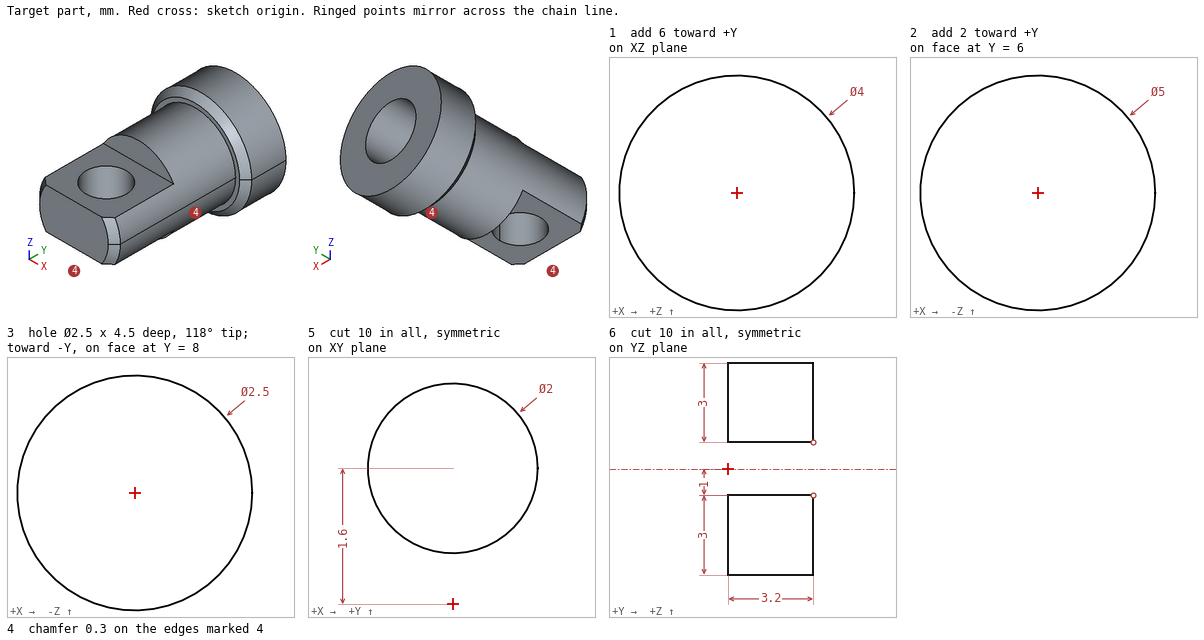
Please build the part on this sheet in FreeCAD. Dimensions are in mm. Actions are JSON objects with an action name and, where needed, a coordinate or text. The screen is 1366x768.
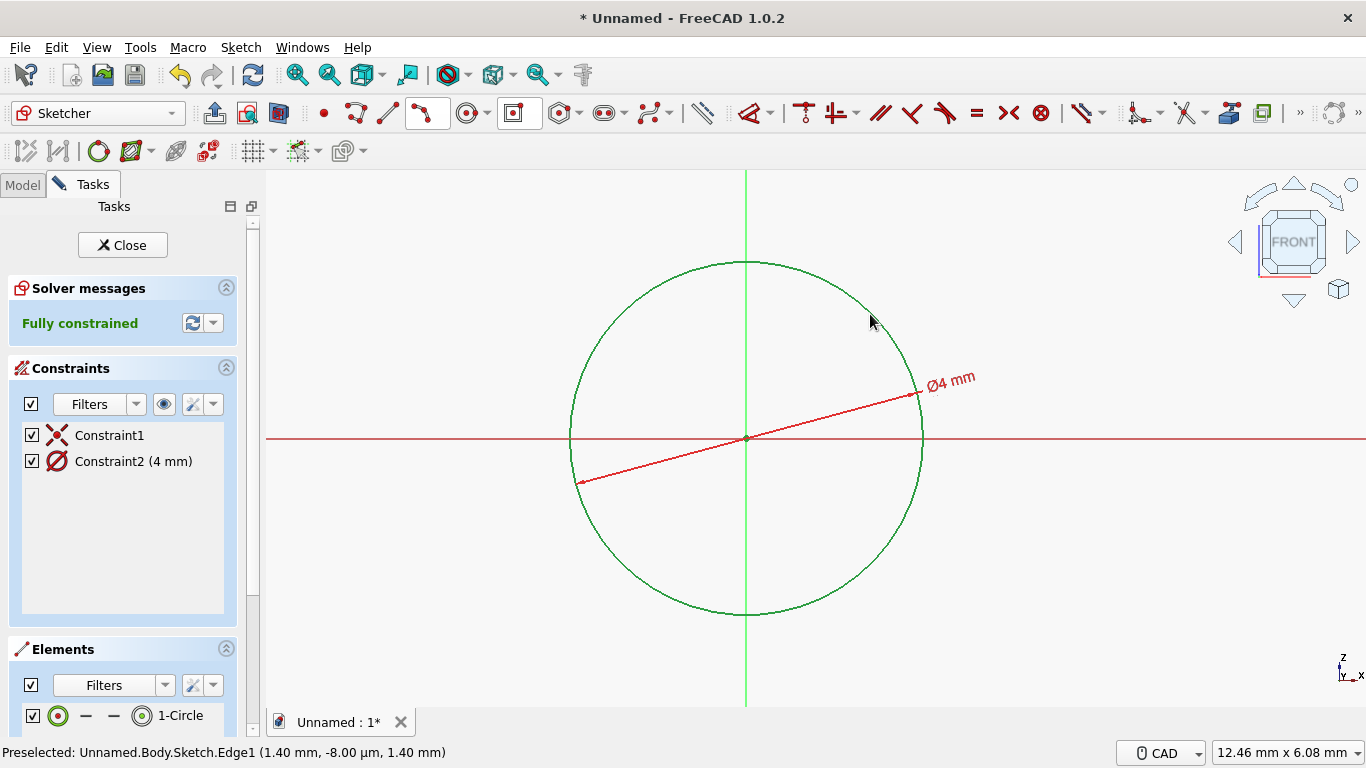
{"action": "left_click", "coordinate": [123, 245]}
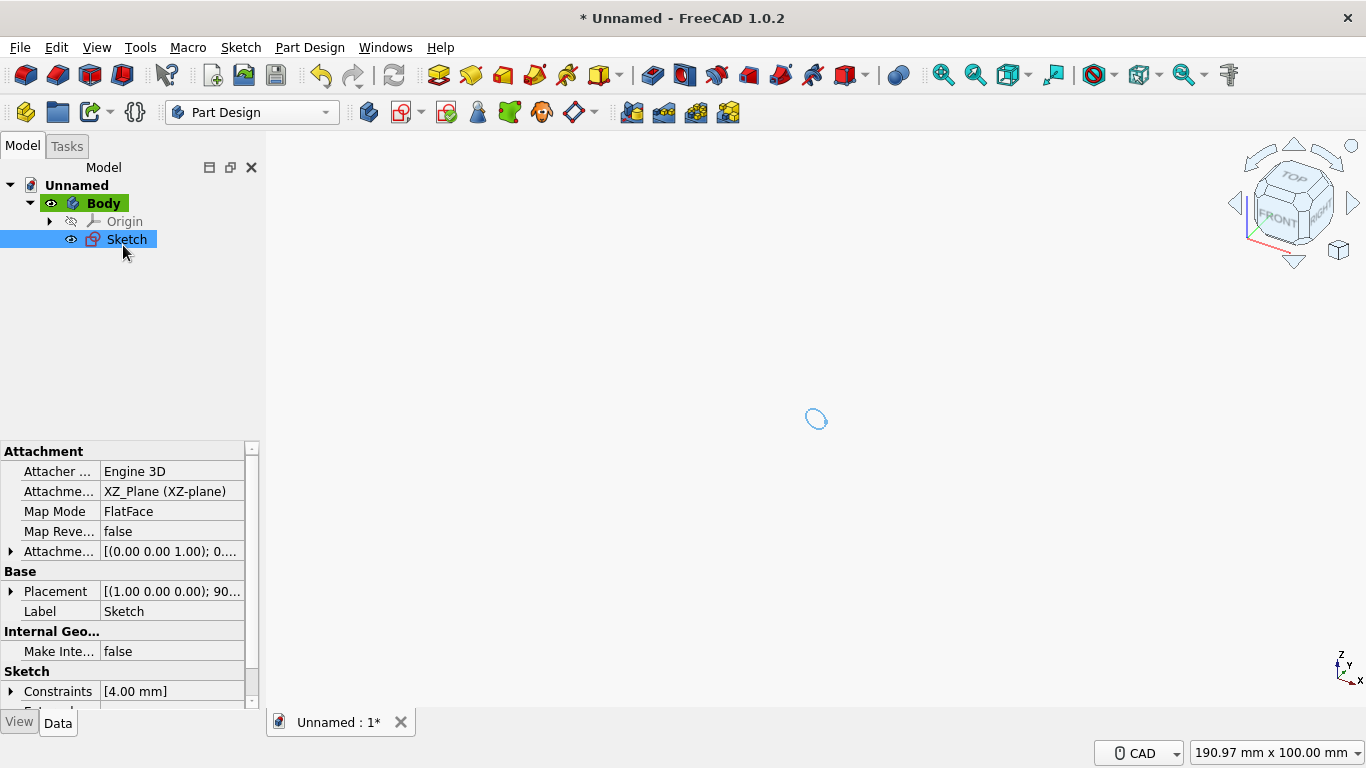
{"action": "left_click", "coordinate": [440, 76]}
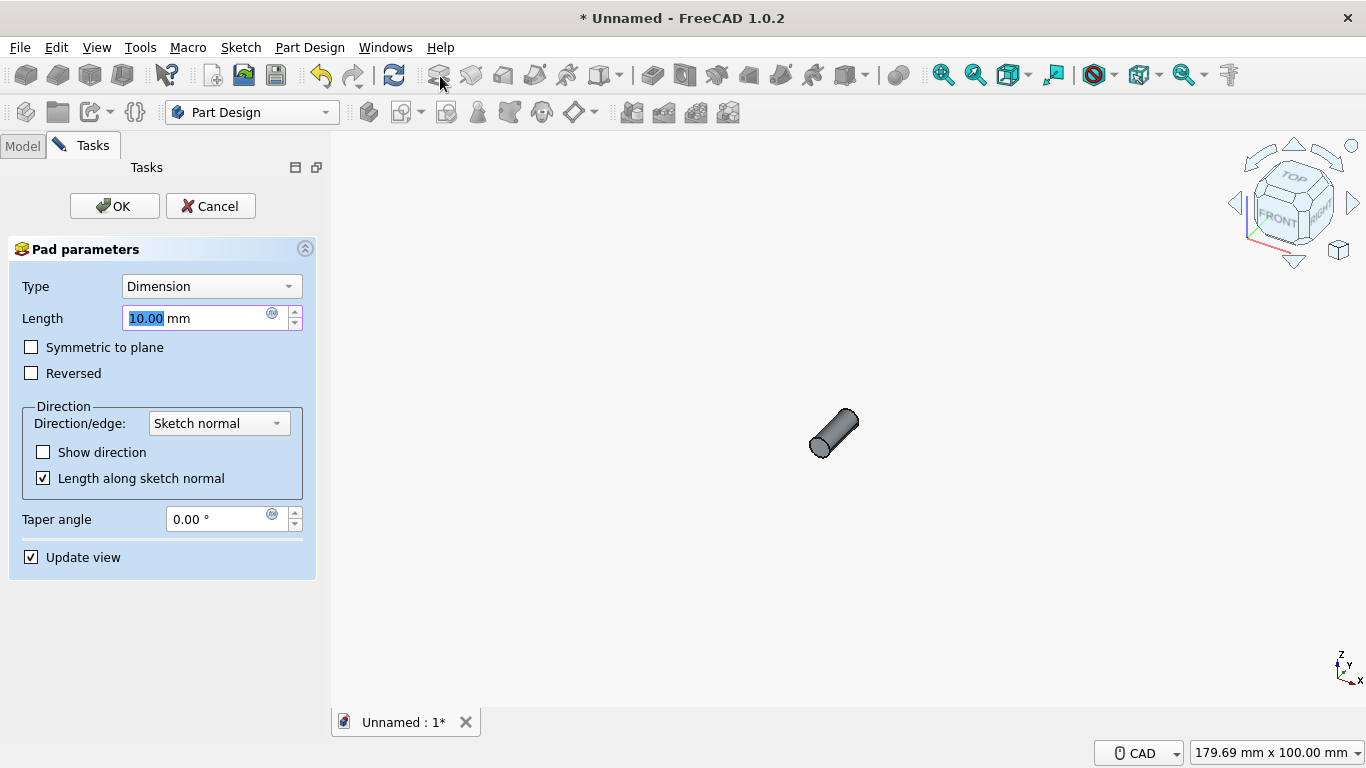
{"action": "type", "text": "6"}
{"action": "key", "text": "Tab"}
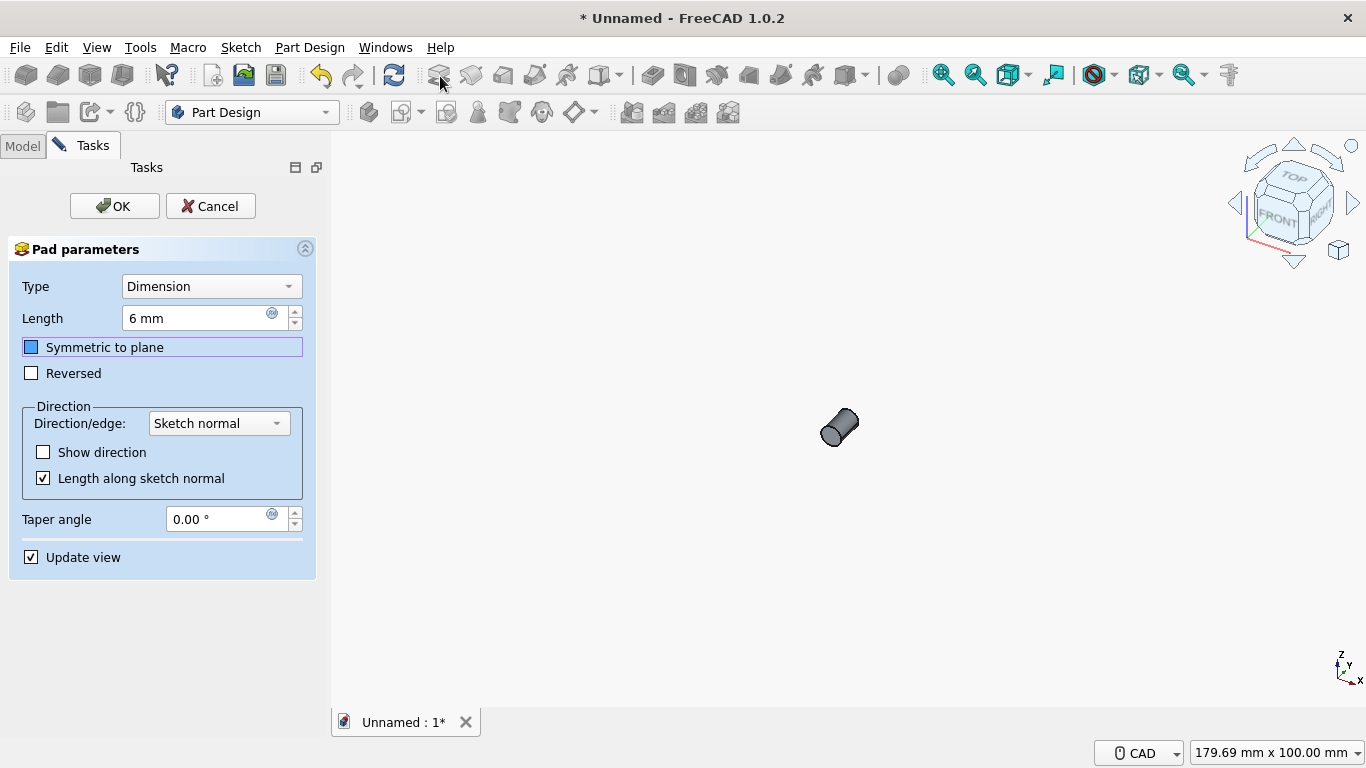
{"action": "left_click", "coordinate": [30, 373]}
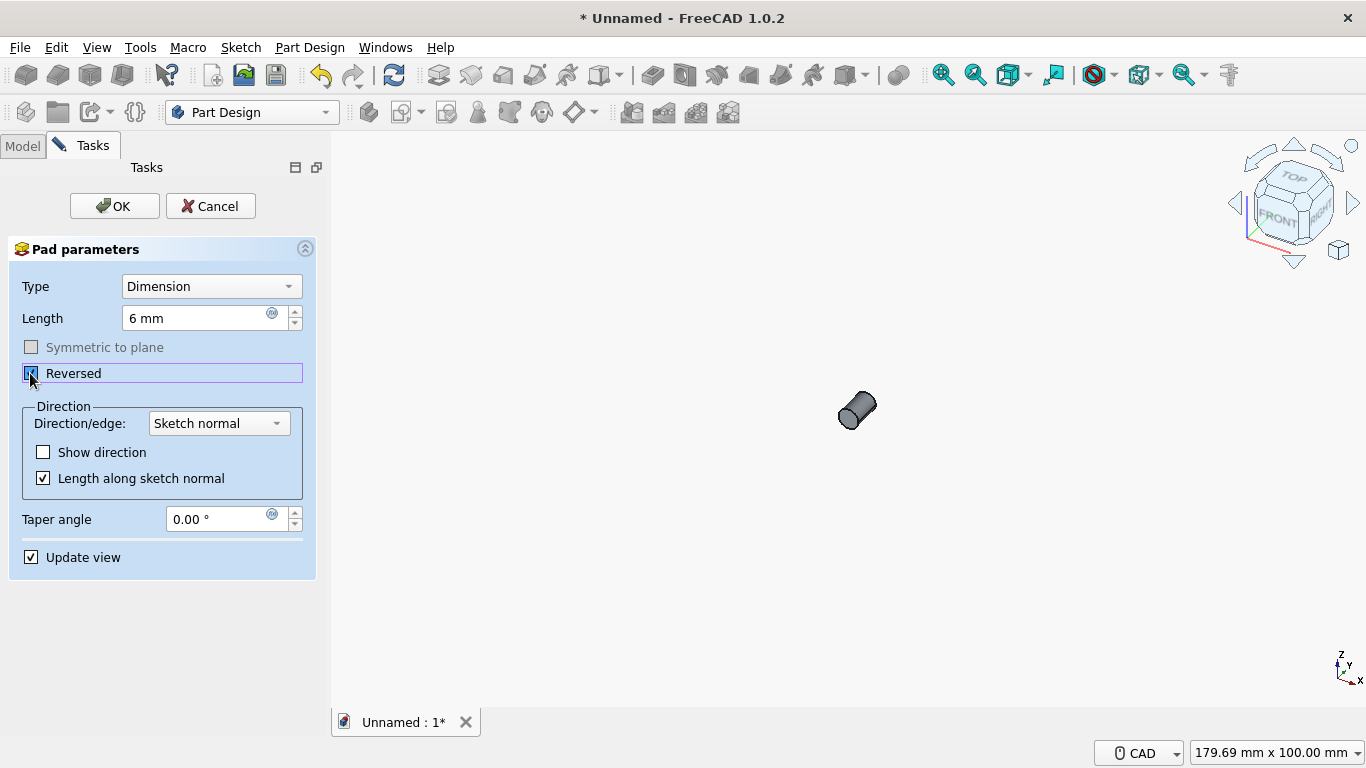
{"action": "left_click", "coordinate": [115, 206]}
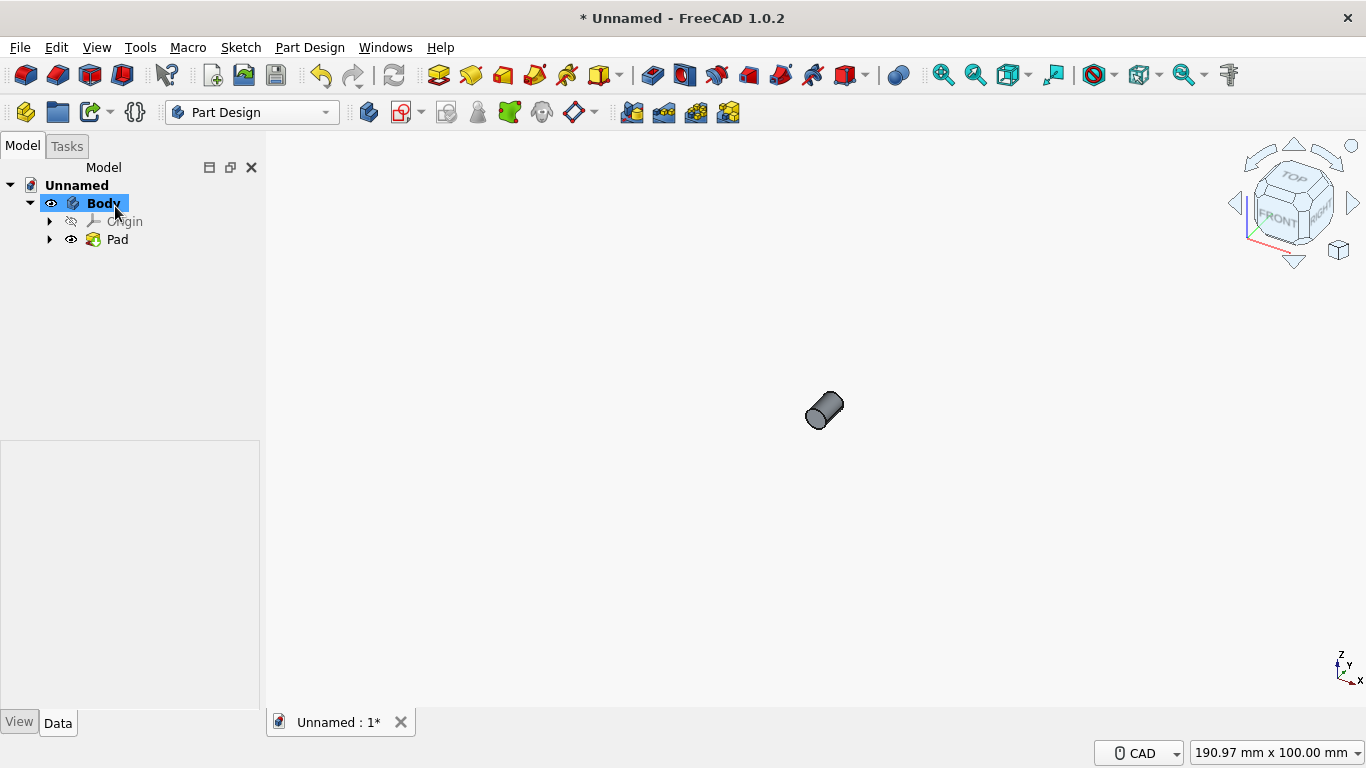
{"action": "key", "text": "v f"}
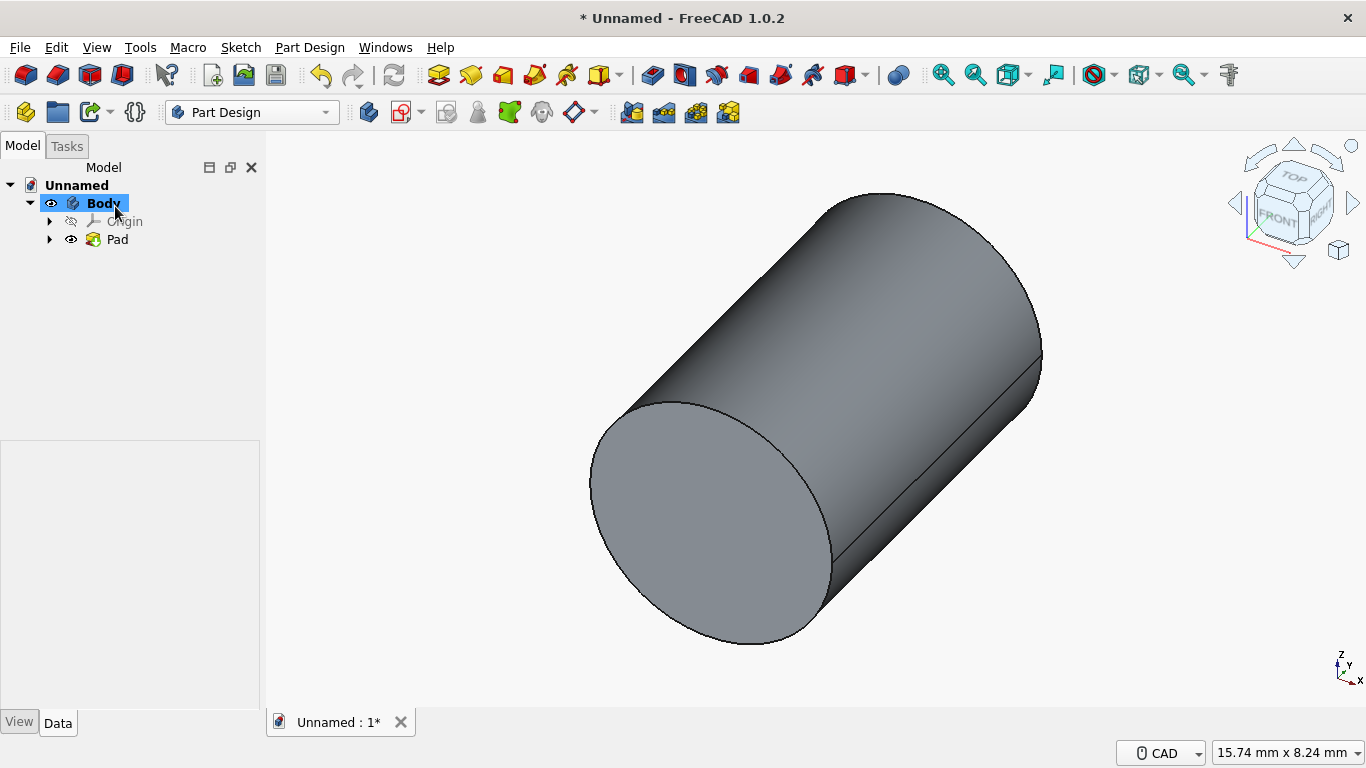
{"action": "key", "text": "4"}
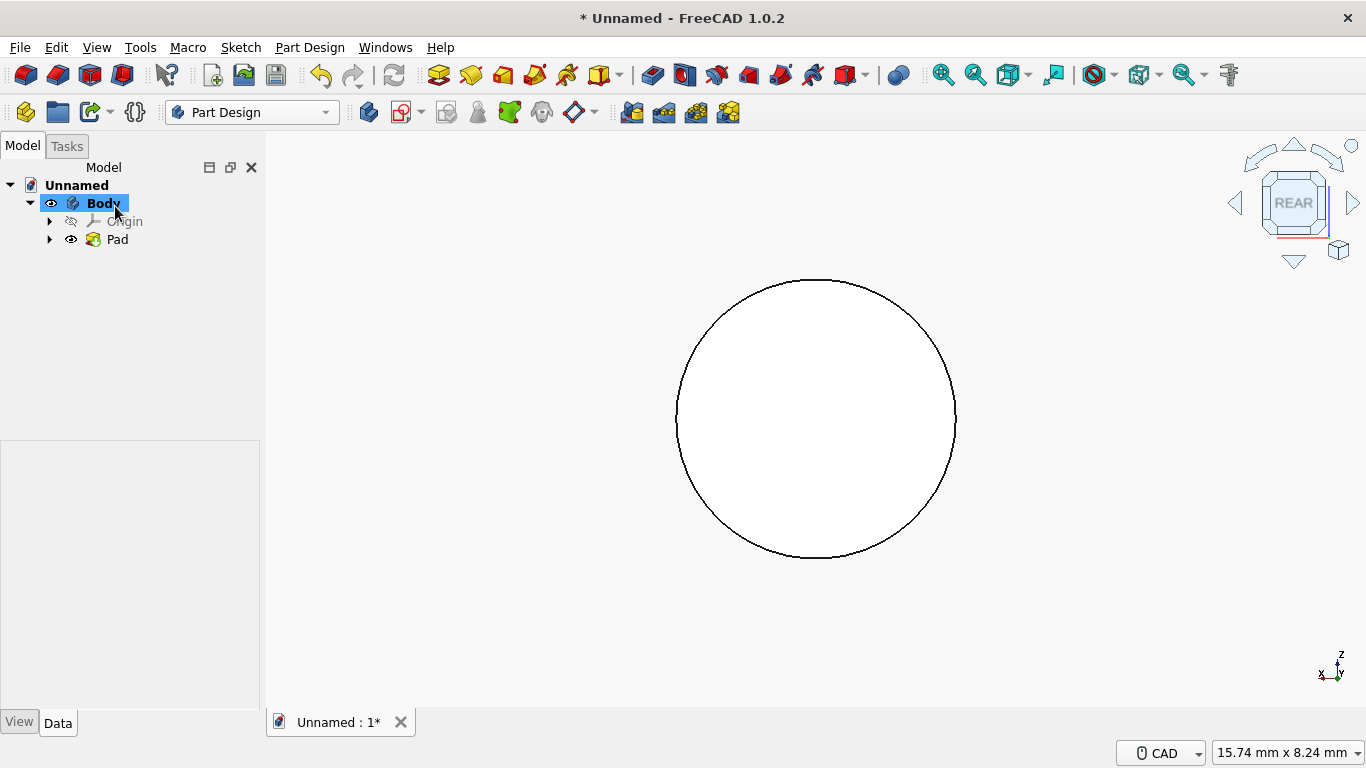
{"action": "left_click", "coordinate": [816, 418]}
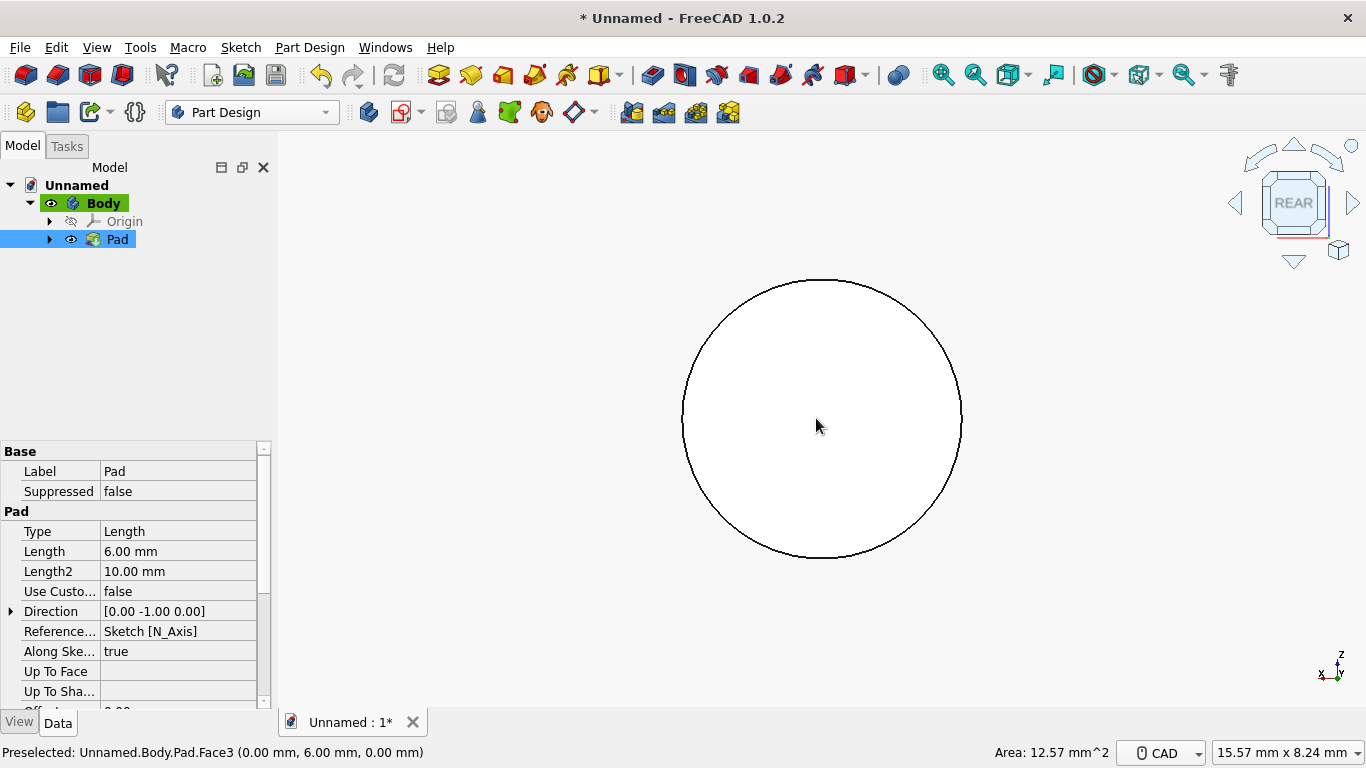
{"action": "left_click", "coordinate": [402, 112]}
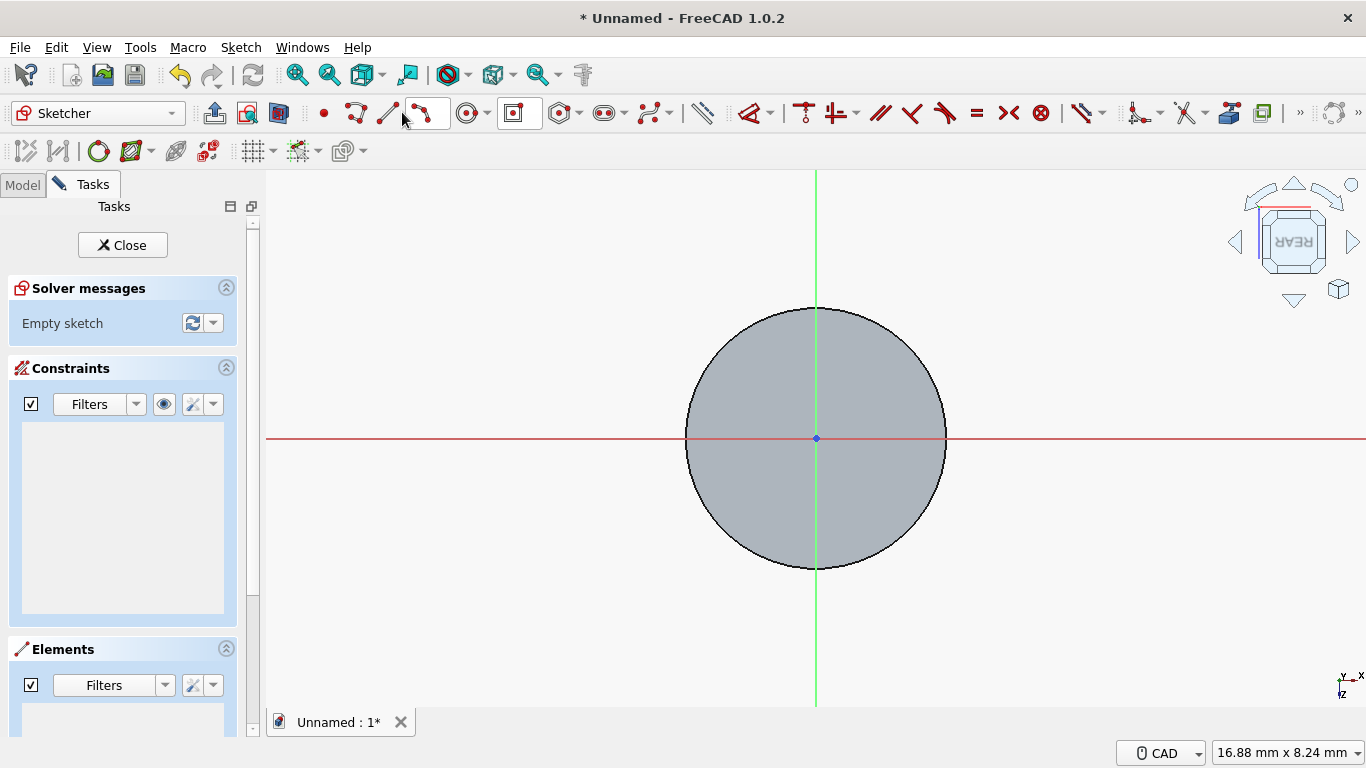
{"action": "left_click", "coordinate": [468, 114]}